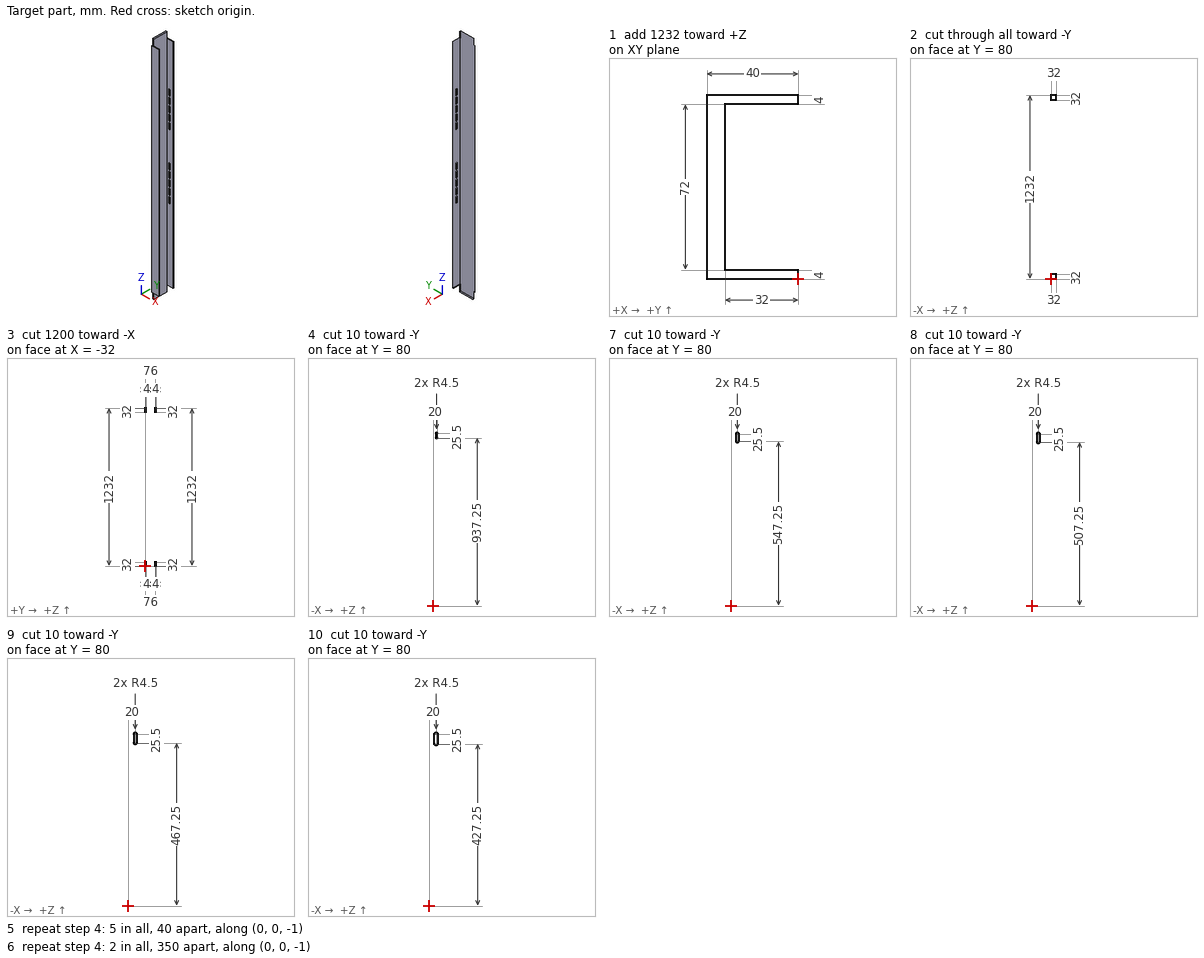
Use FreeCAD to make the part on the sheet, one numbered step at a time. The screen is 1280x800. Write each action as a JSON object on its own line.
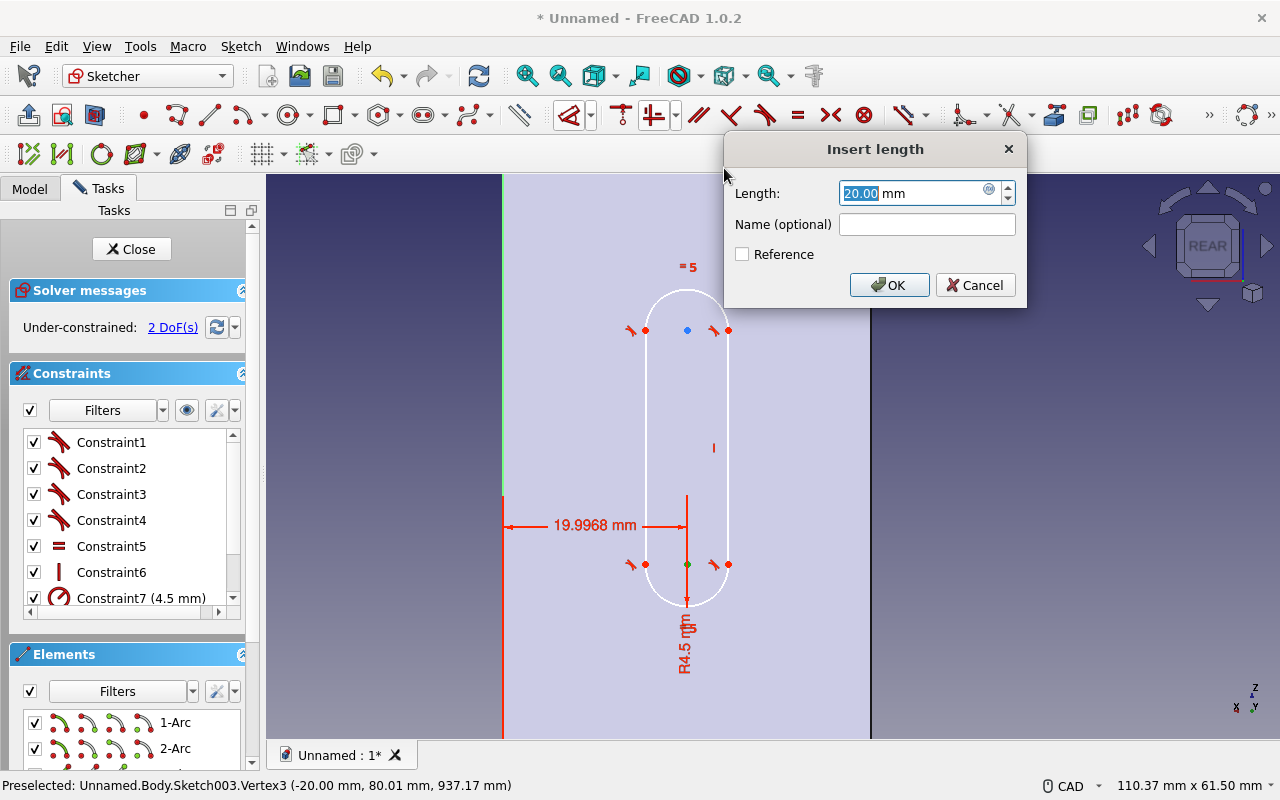
{"action": "type", "text": "20"}
{"action": "key", "text": "Return"}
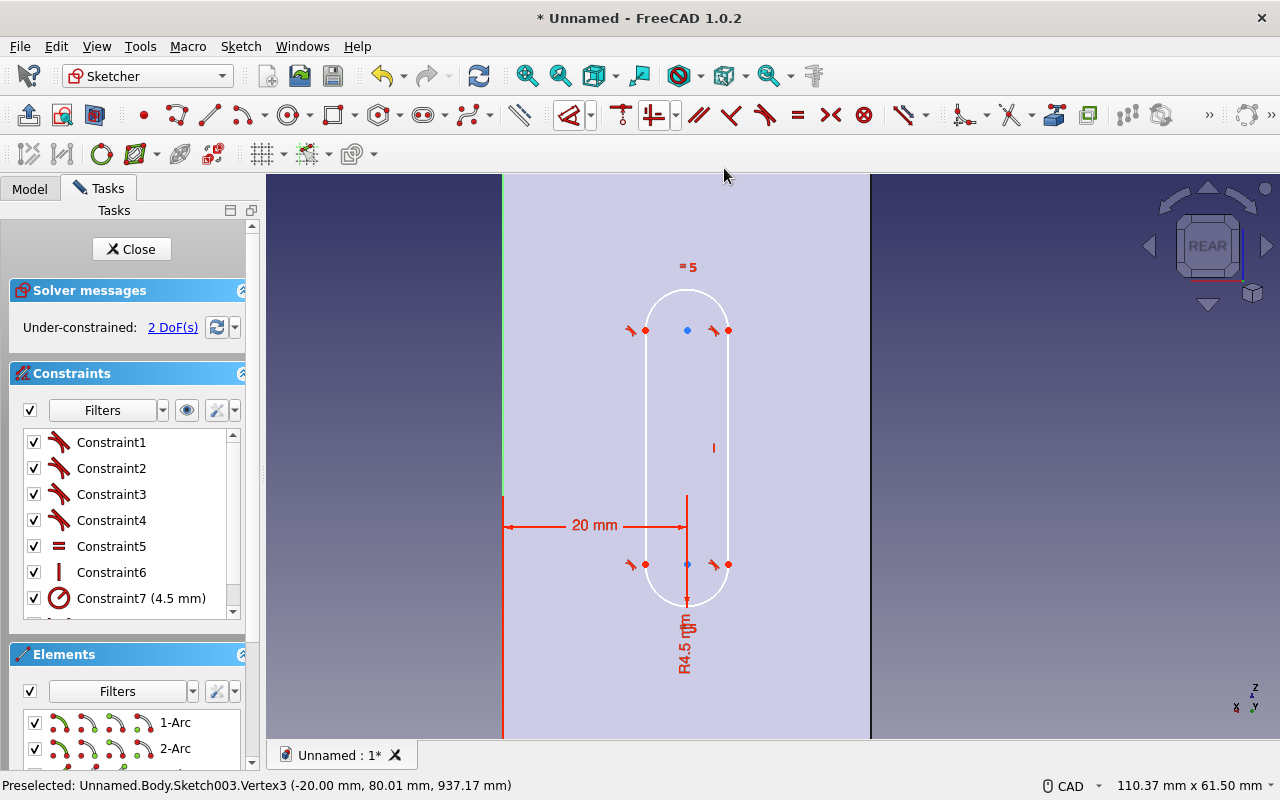
{"action": "left_click", "coordinate": [646, 495]}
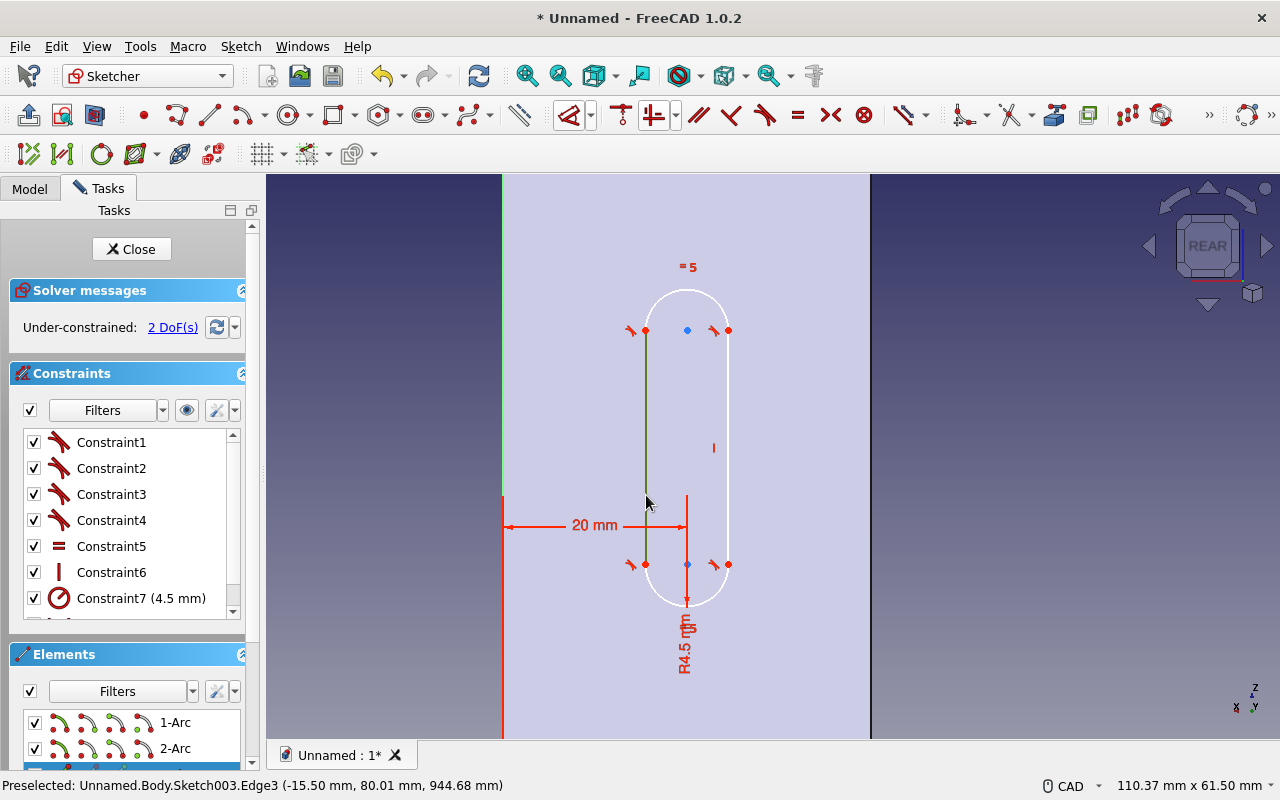
{"action": "left_click", "coordinate": [590, 116]}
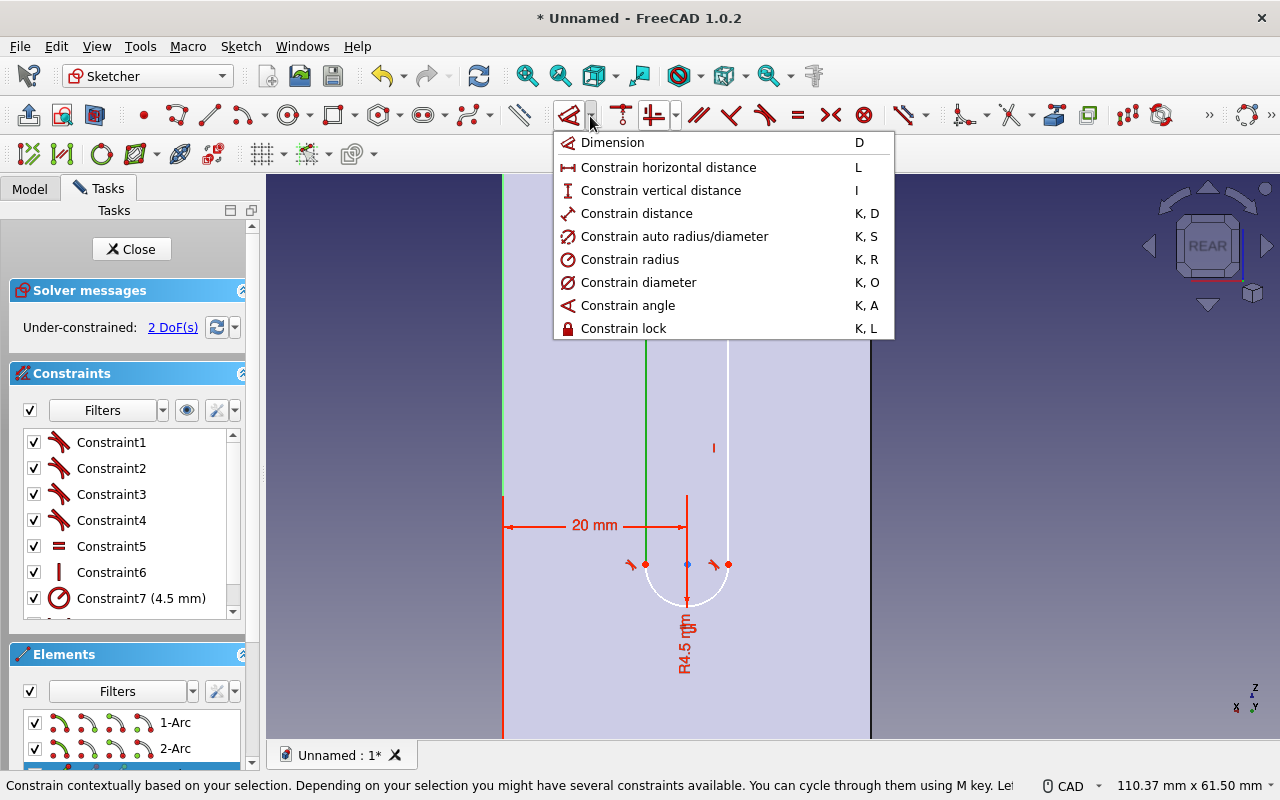
{"action": "left_click", "coordinate": [724, 190]}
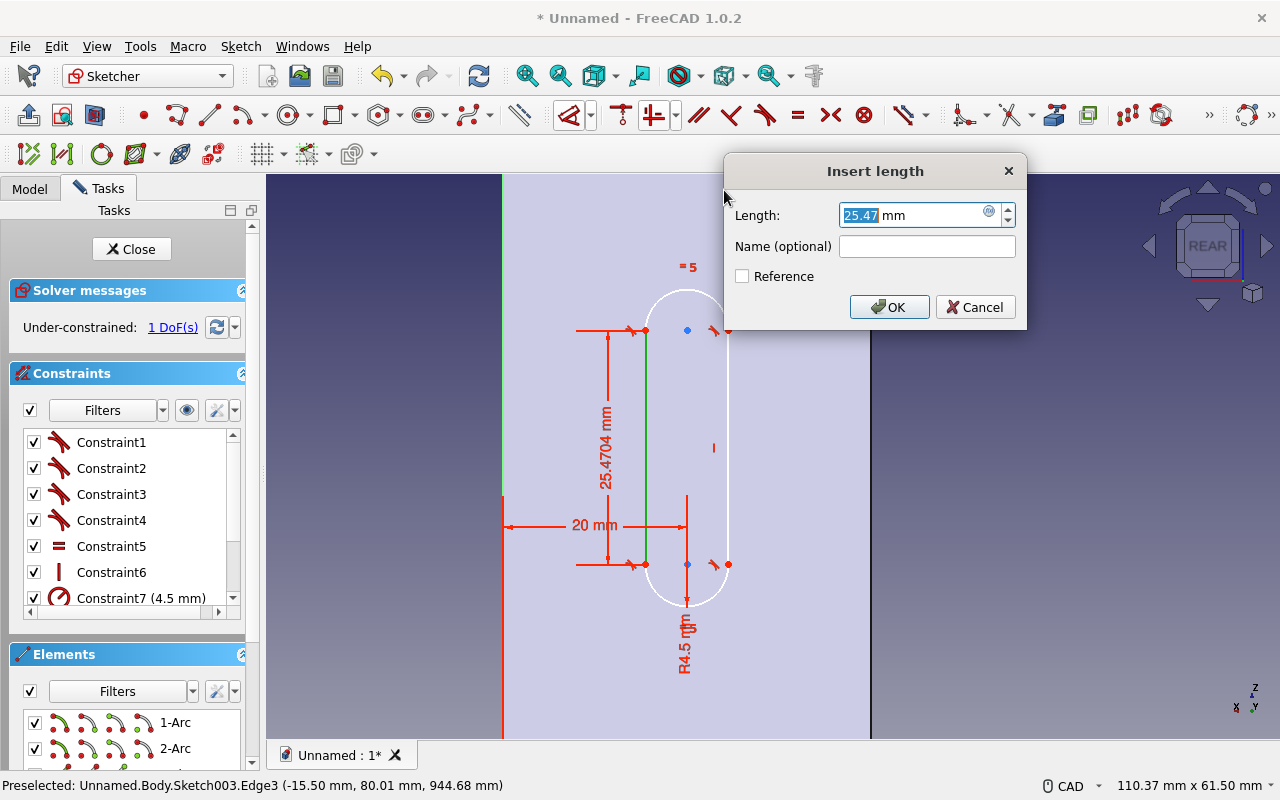
{"action": "type", "text": "25.5"}
{"action": "key", "text": "Return"}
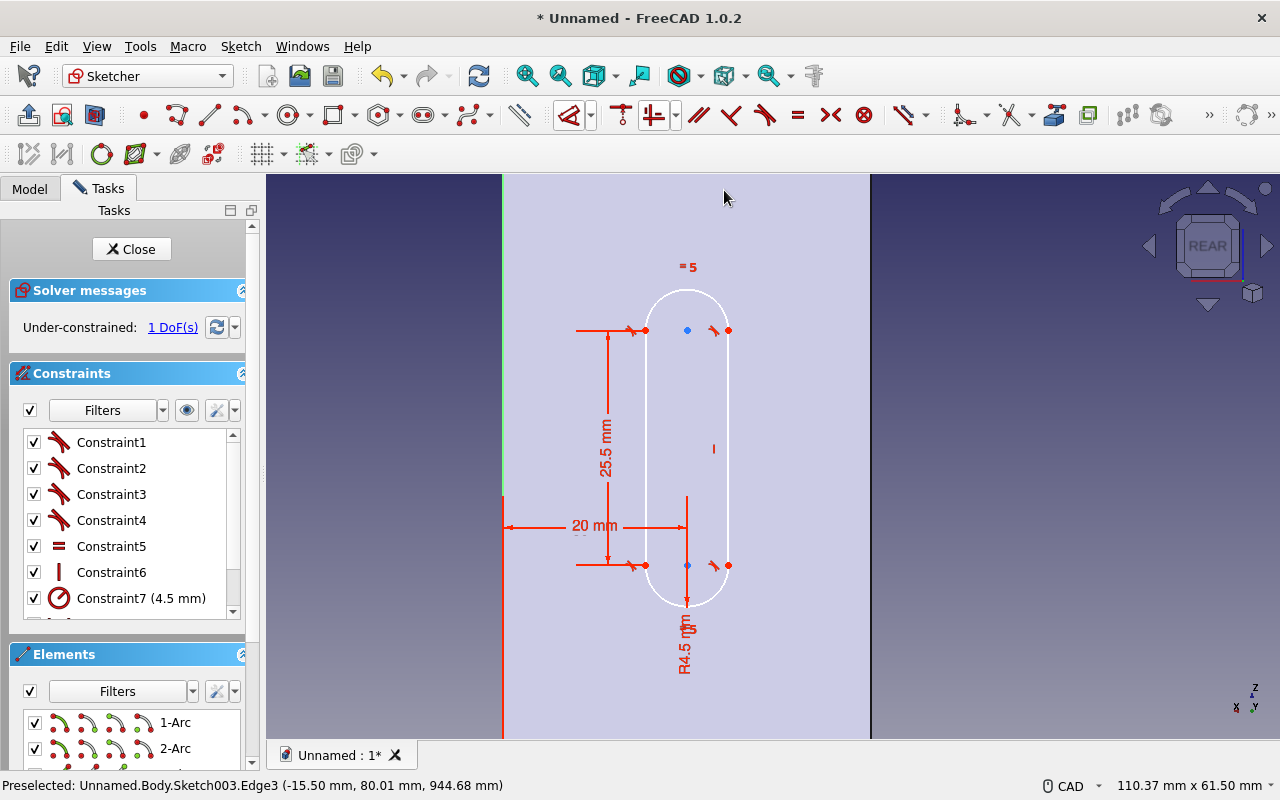
{"action": "left_click", "coordinate": [646, 565]}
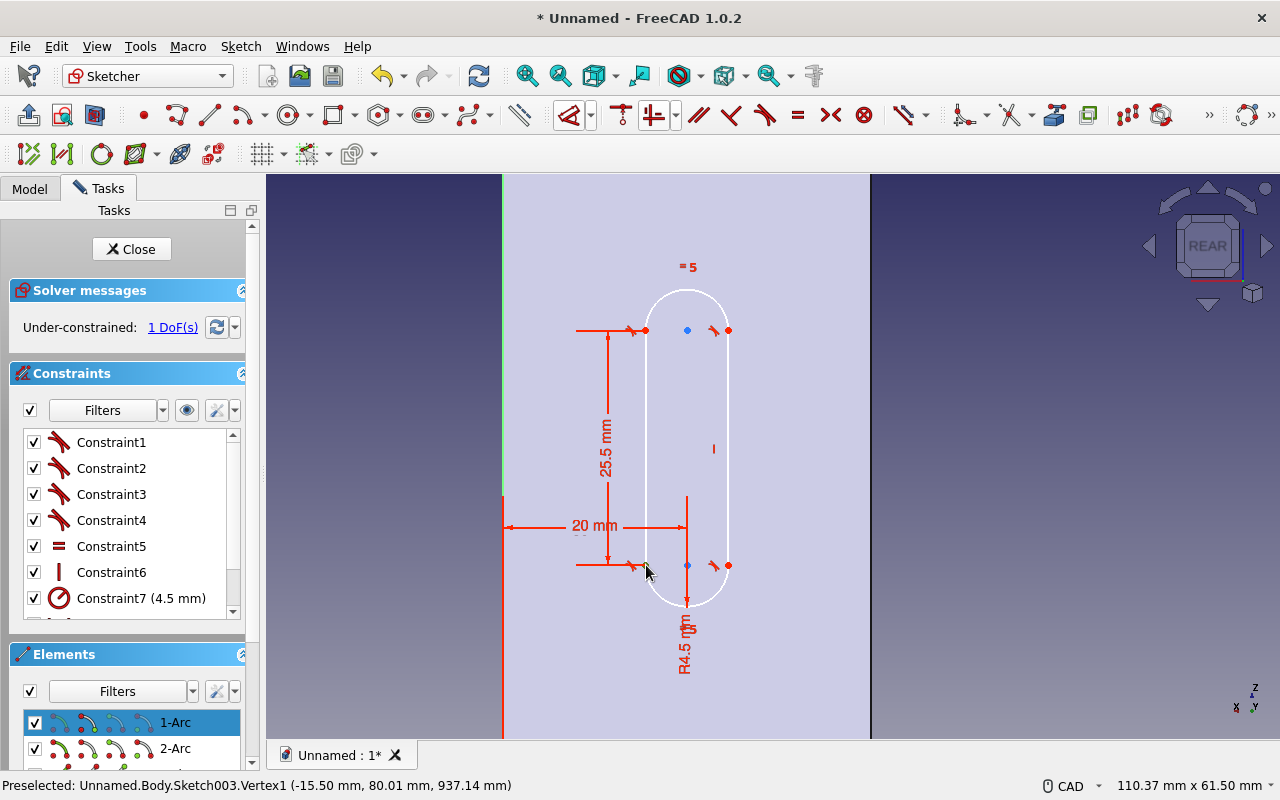
{"action": "key", "text": "i"}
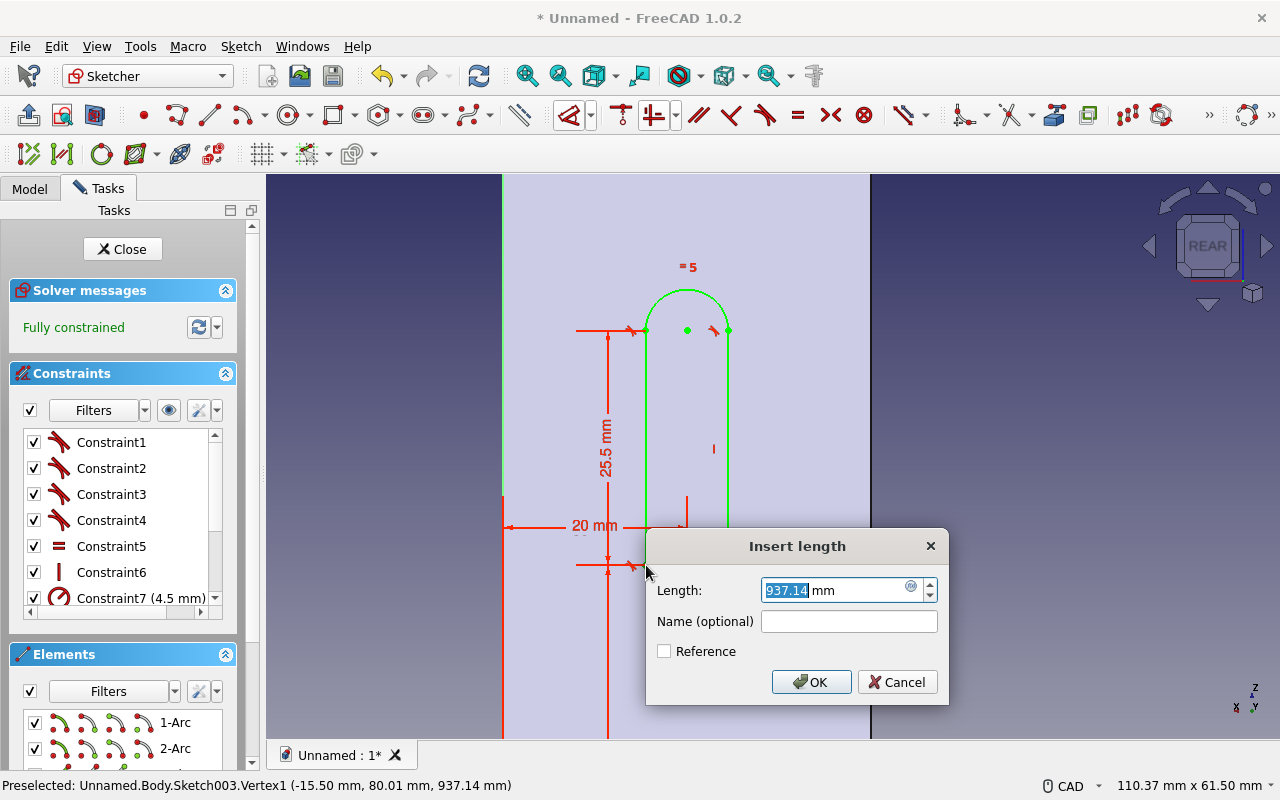
{"action": "type", "text": "937.25"}
{"action": "key", "text": "Return"}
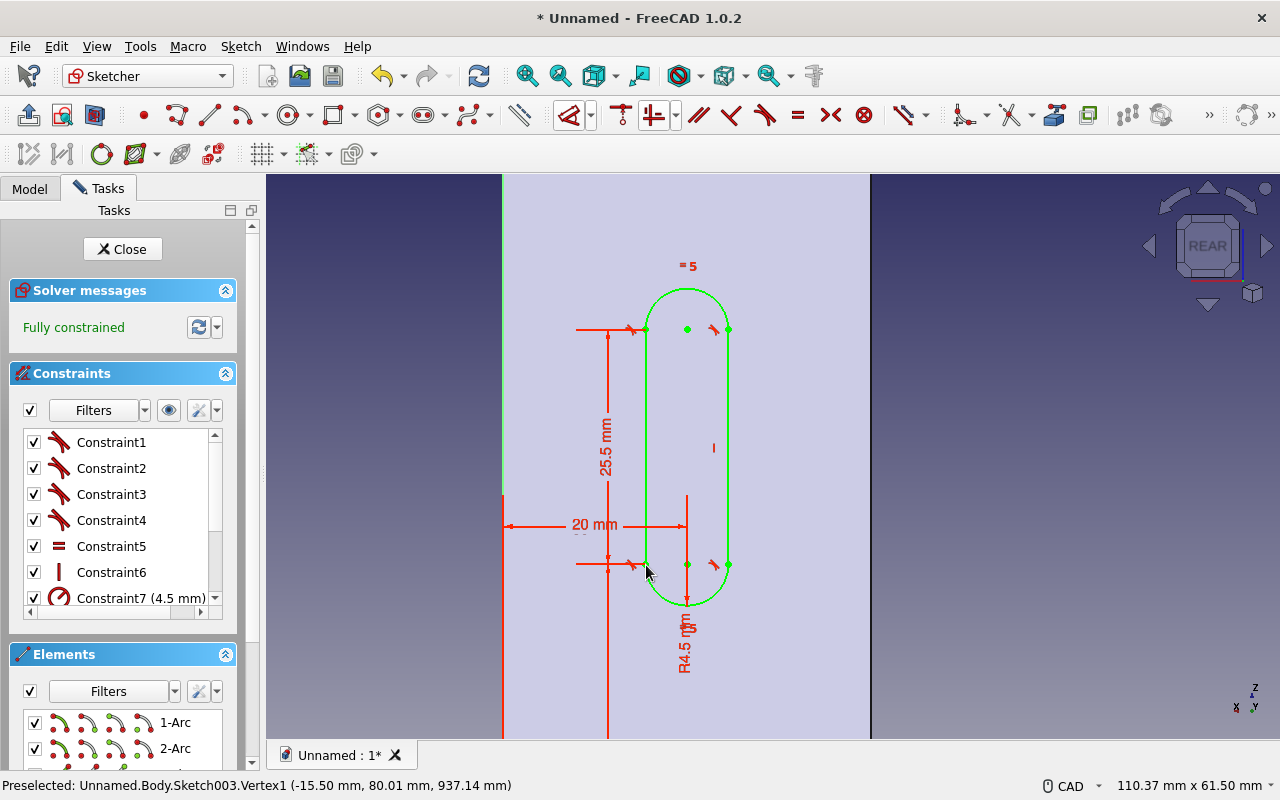
{"action": "left_click", "coordinate": [123, 249]}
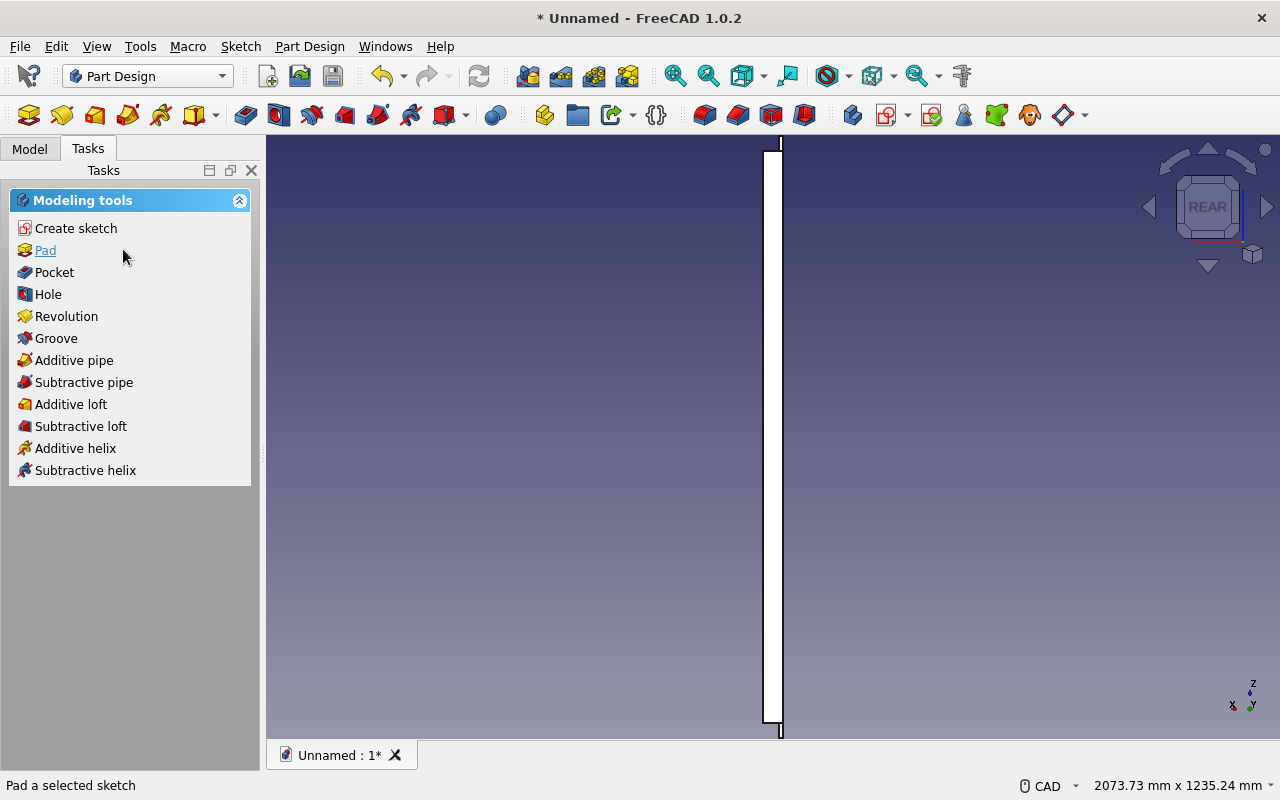
{"action": "left_click", "coordinate": [246, 116]}